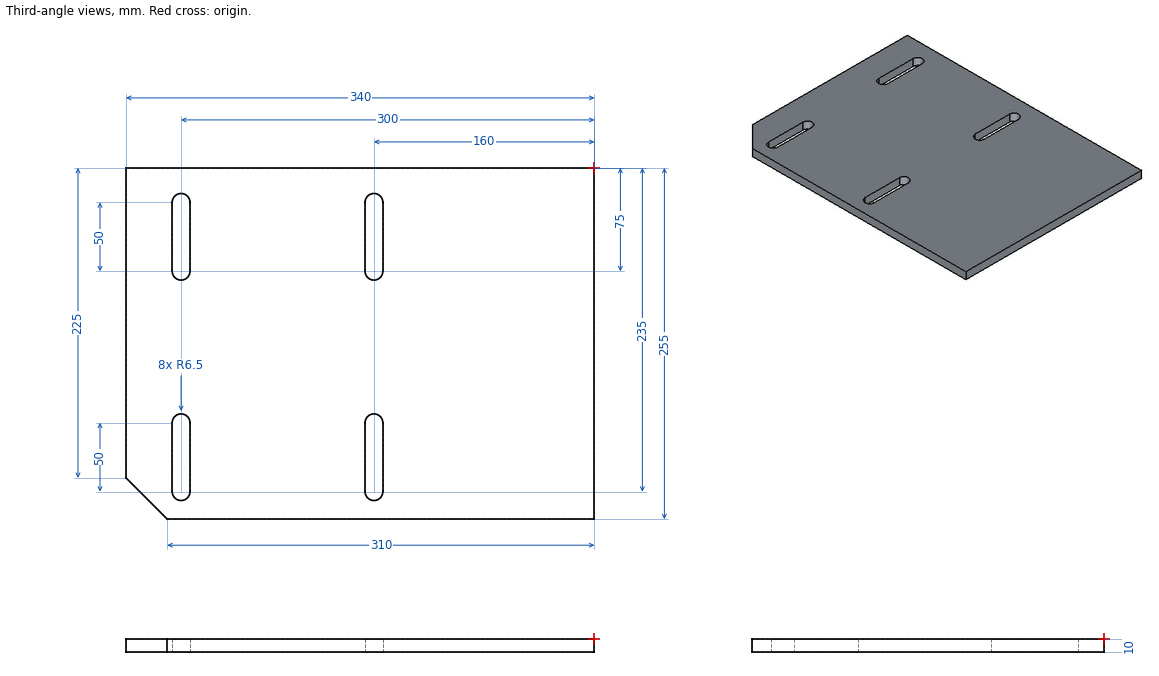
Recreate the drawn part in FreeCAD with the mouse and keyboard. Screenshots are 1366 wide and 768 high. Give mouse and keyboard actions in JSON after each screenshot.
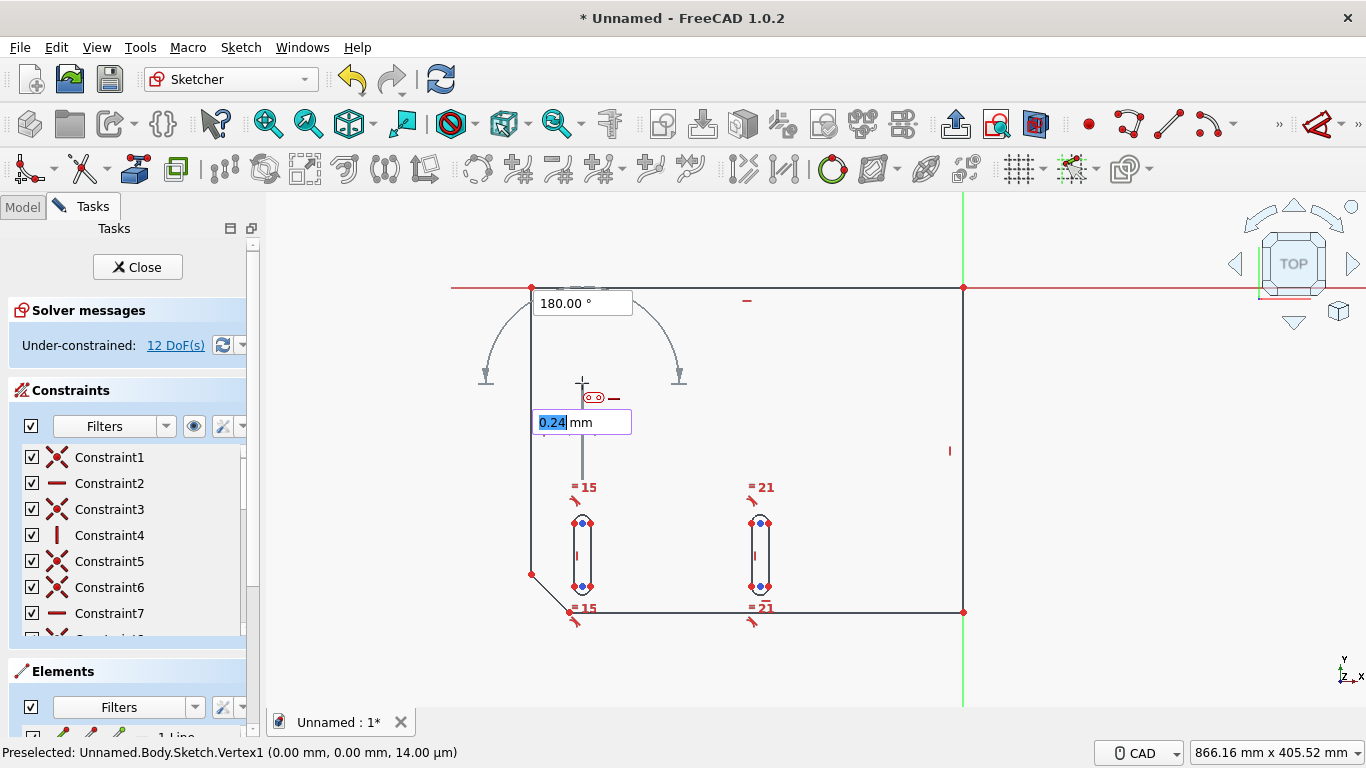
{"action": "left_click", "coordinate": [583, 320]}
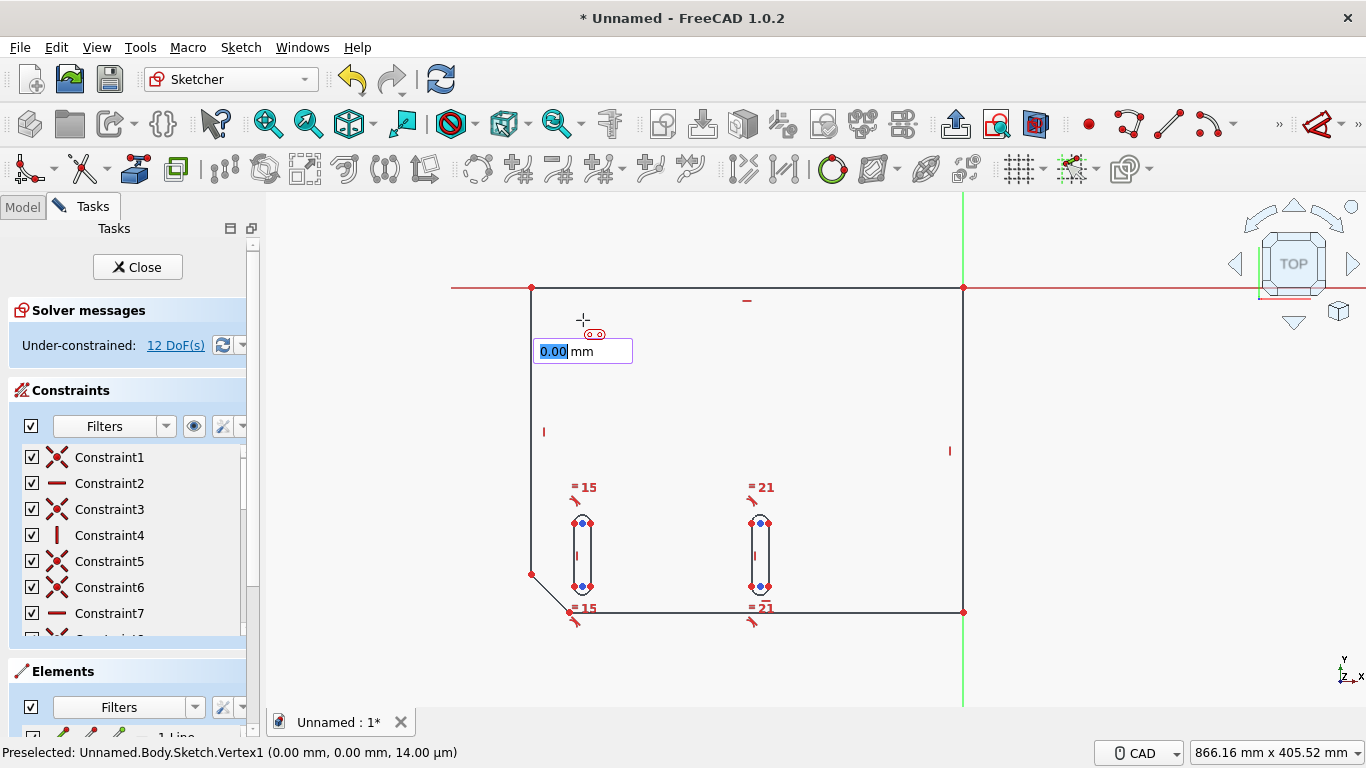
{"action": "scroll", "coordinate": [591, 351], "scroll_direction": "up", "scroll_amount": 4}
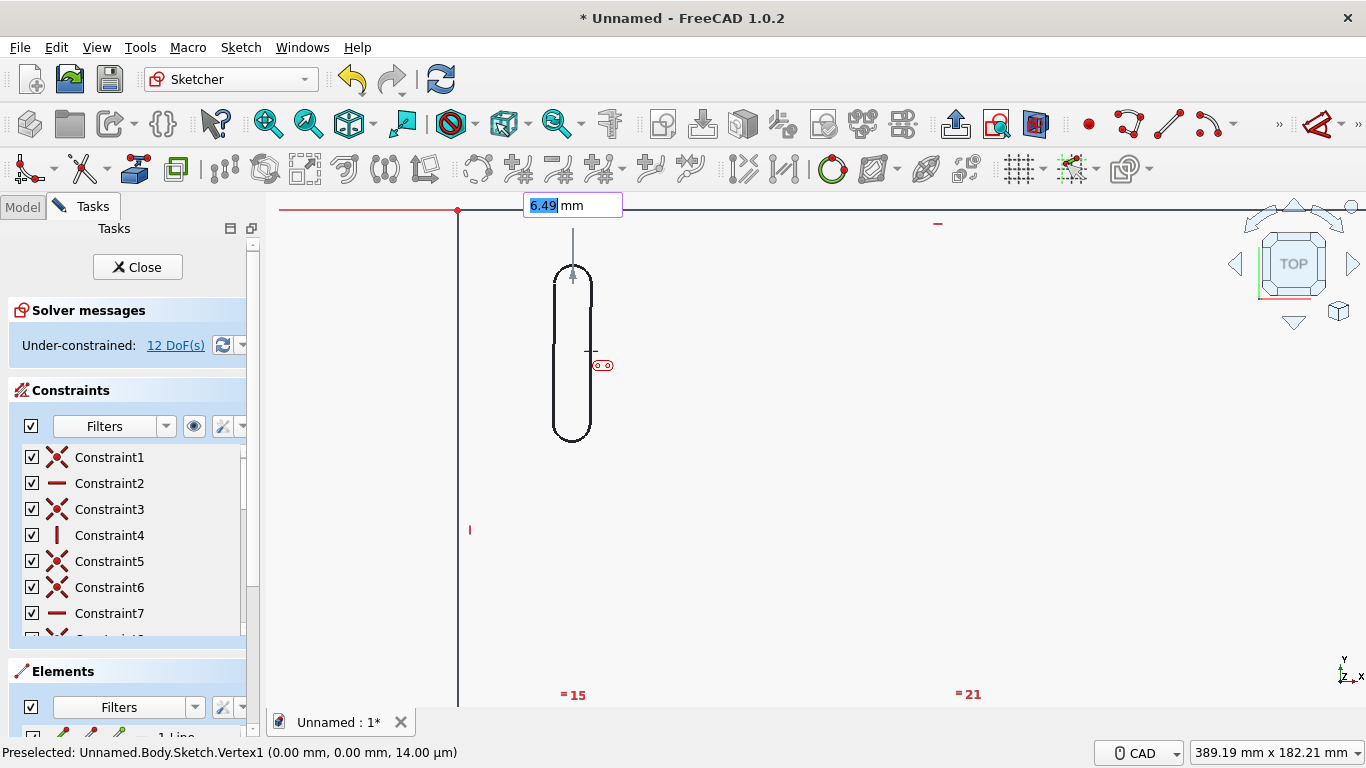
{"action": "left_click", "coordinate": [590, 352]}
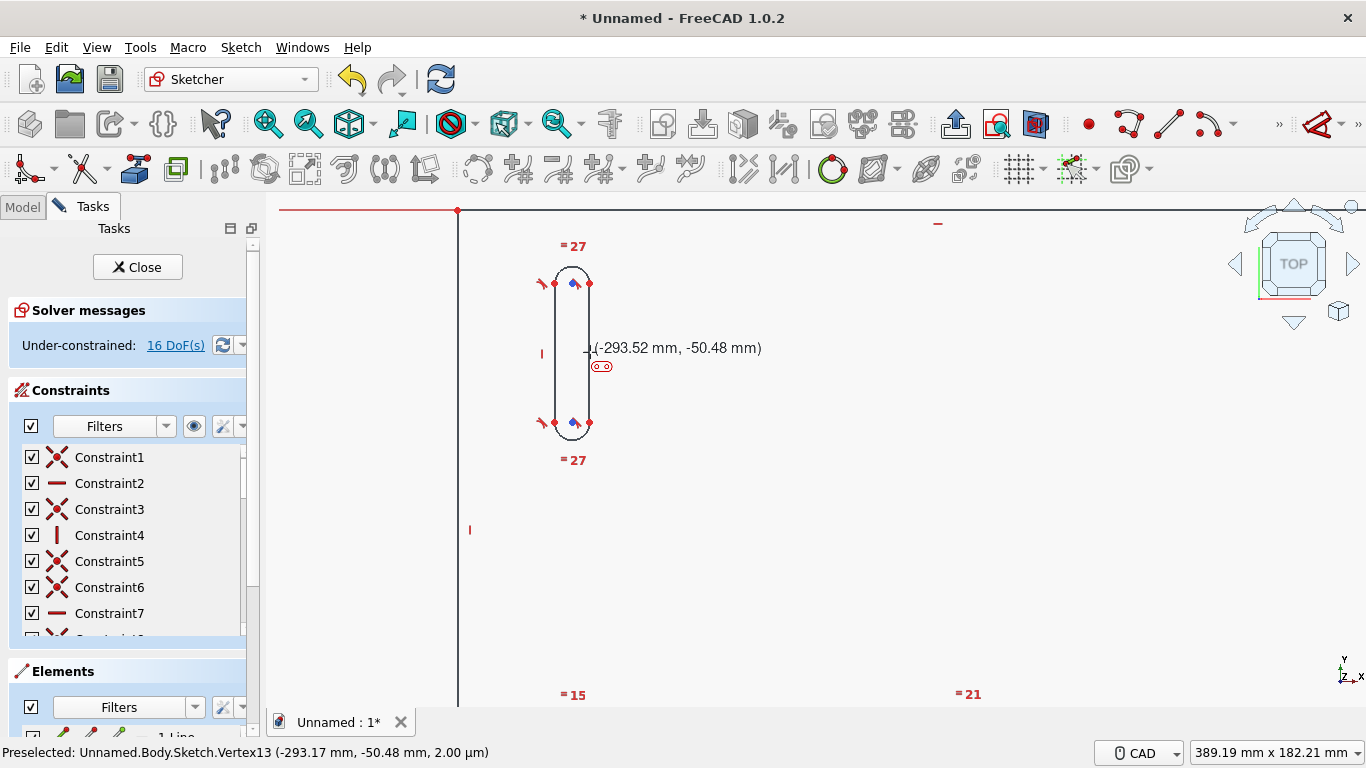
{"action": "scroll", "coordinate": [967, 422], "scroll_direction": "up", "scroll_amount": 2}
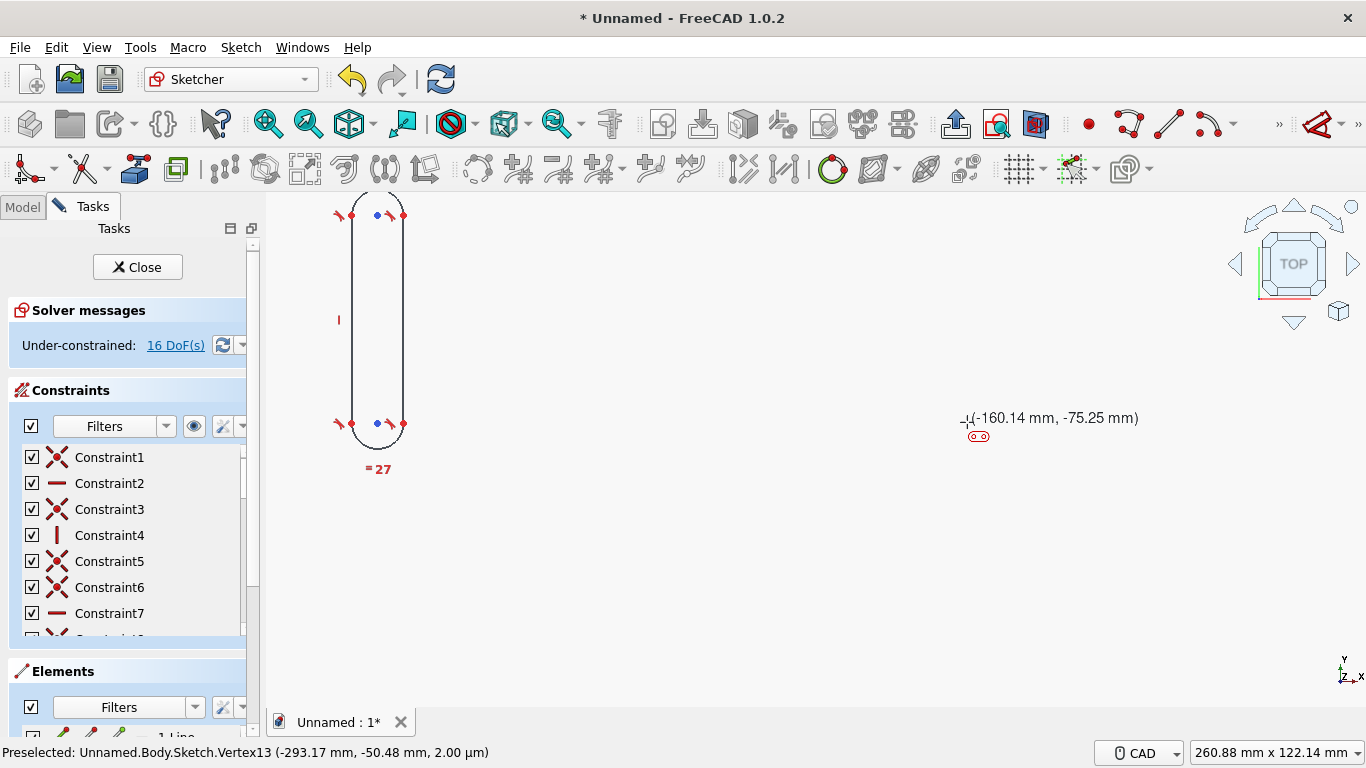
{"action": "left_click", "coordinate": [967, 422]}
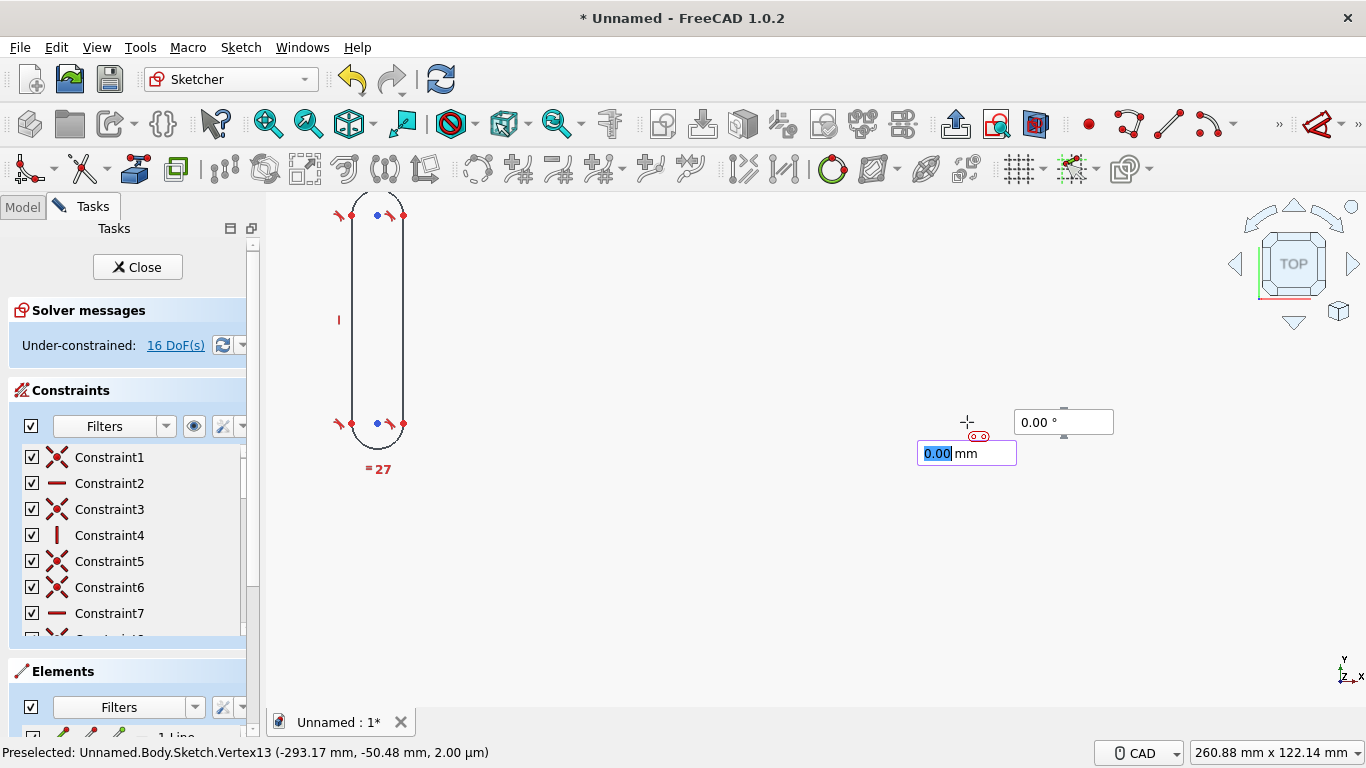
{"action": "scroll", "coordinate": [671, 366], "scroll_direction": "down", "scroll_amount": 6}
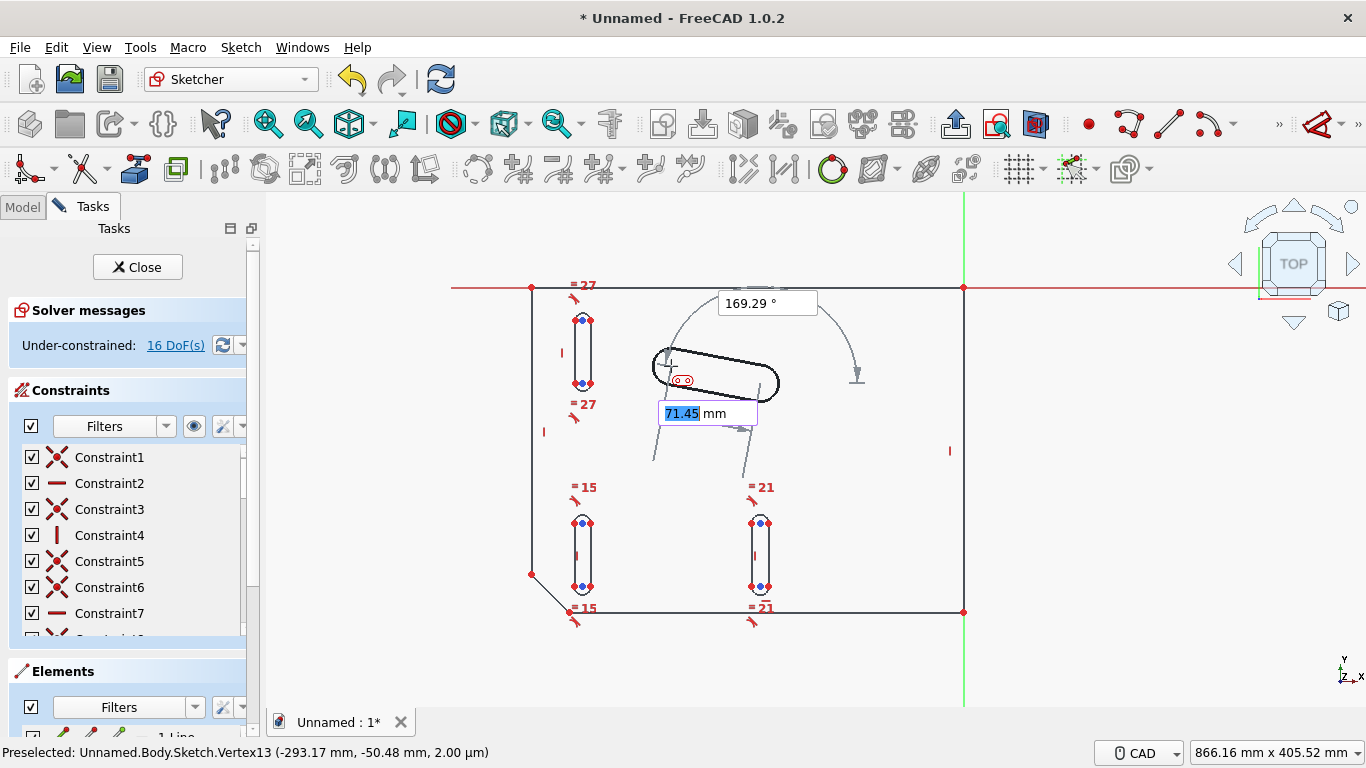
{"action": "left_click", "coordinate": [760, 320]}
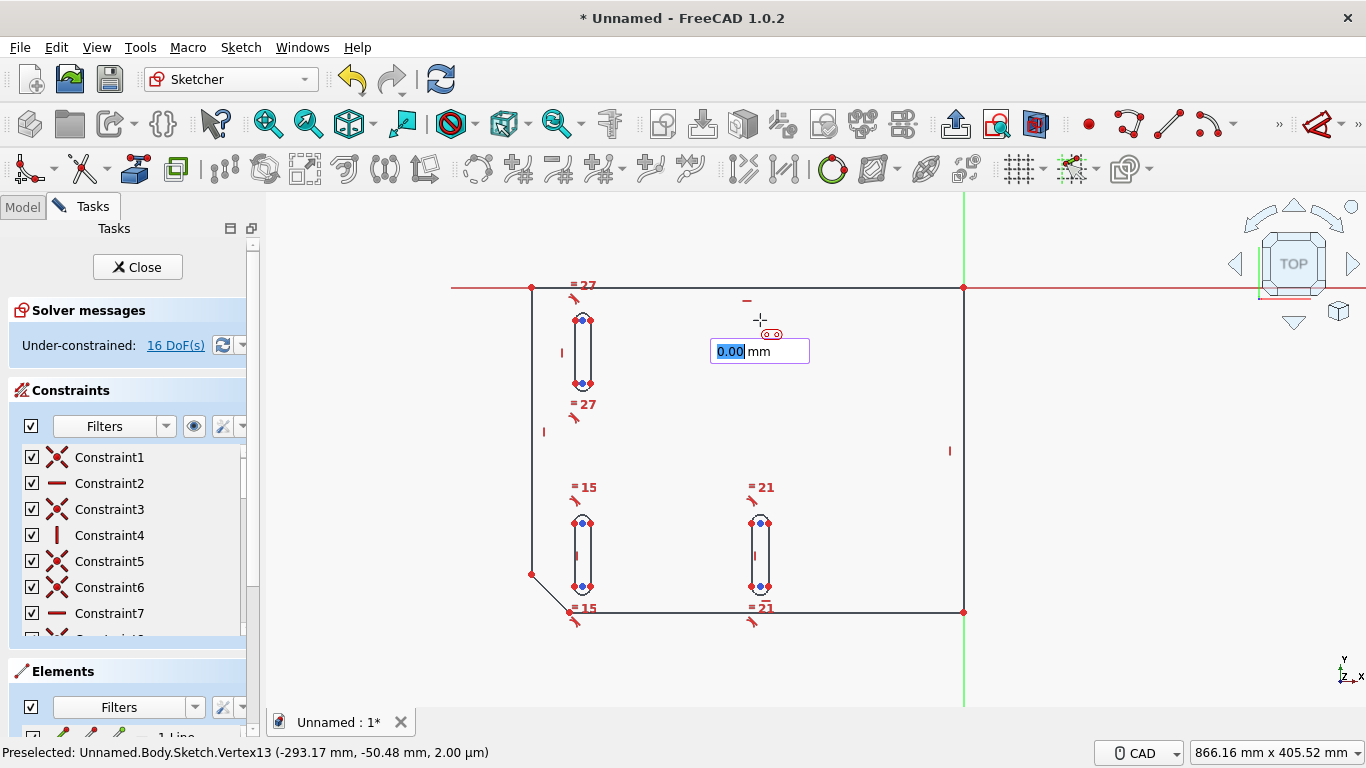
{"action": "scroll", "coordinate": [769, 351], "scroll_direction": "up", "scroll_amount": 4}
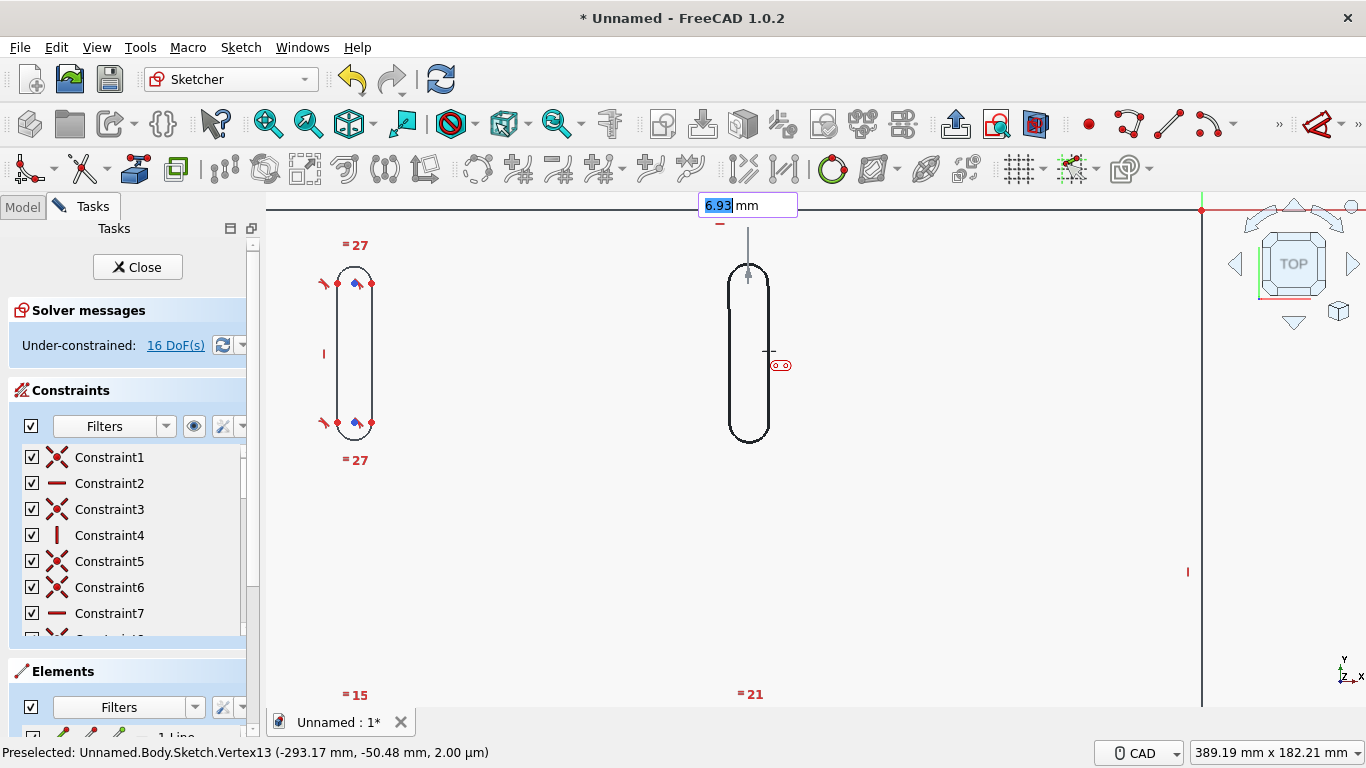
{"action": "left_click", "coordinate": [768, 352]}
{"action": "key", "text": "Escape"}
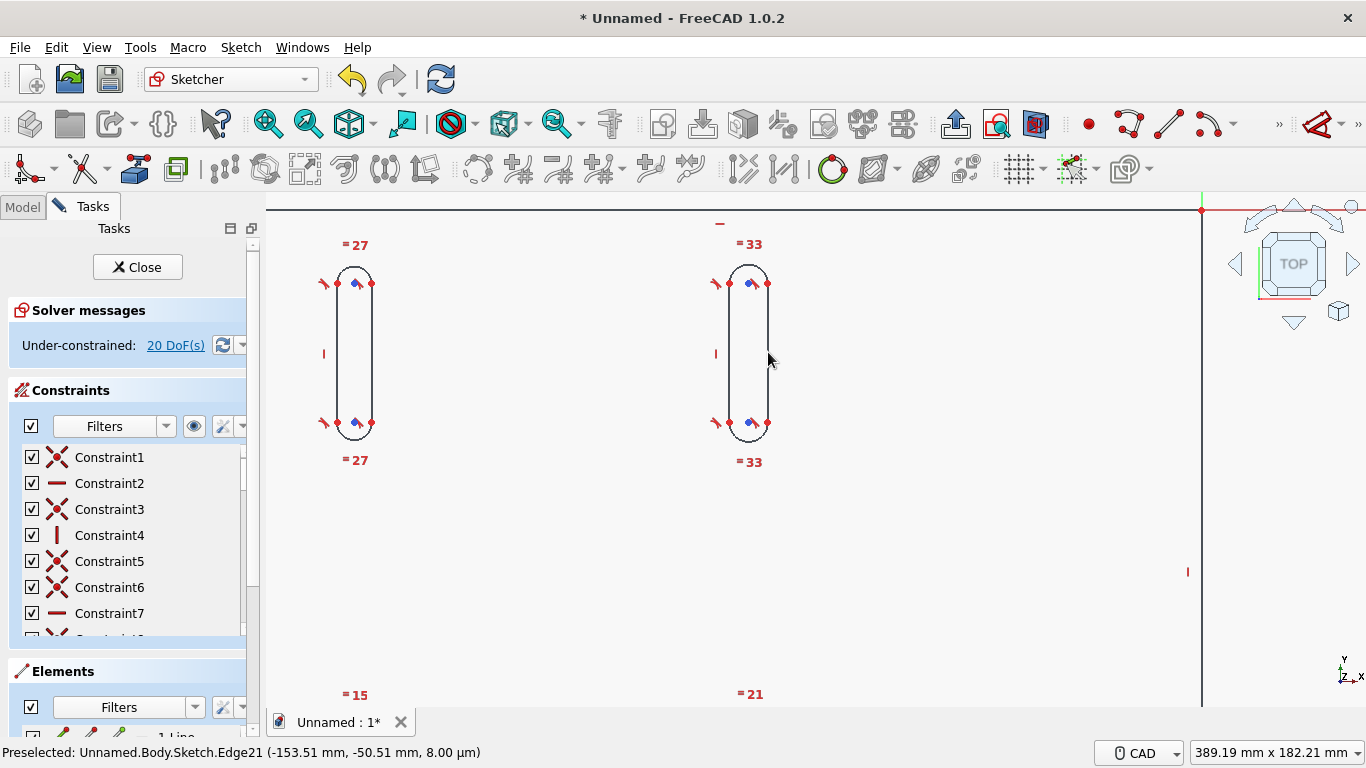
{"action": "scroll", "coordinate": [769, 351], "scroll_direction": "down", "scroll_amount": 4}